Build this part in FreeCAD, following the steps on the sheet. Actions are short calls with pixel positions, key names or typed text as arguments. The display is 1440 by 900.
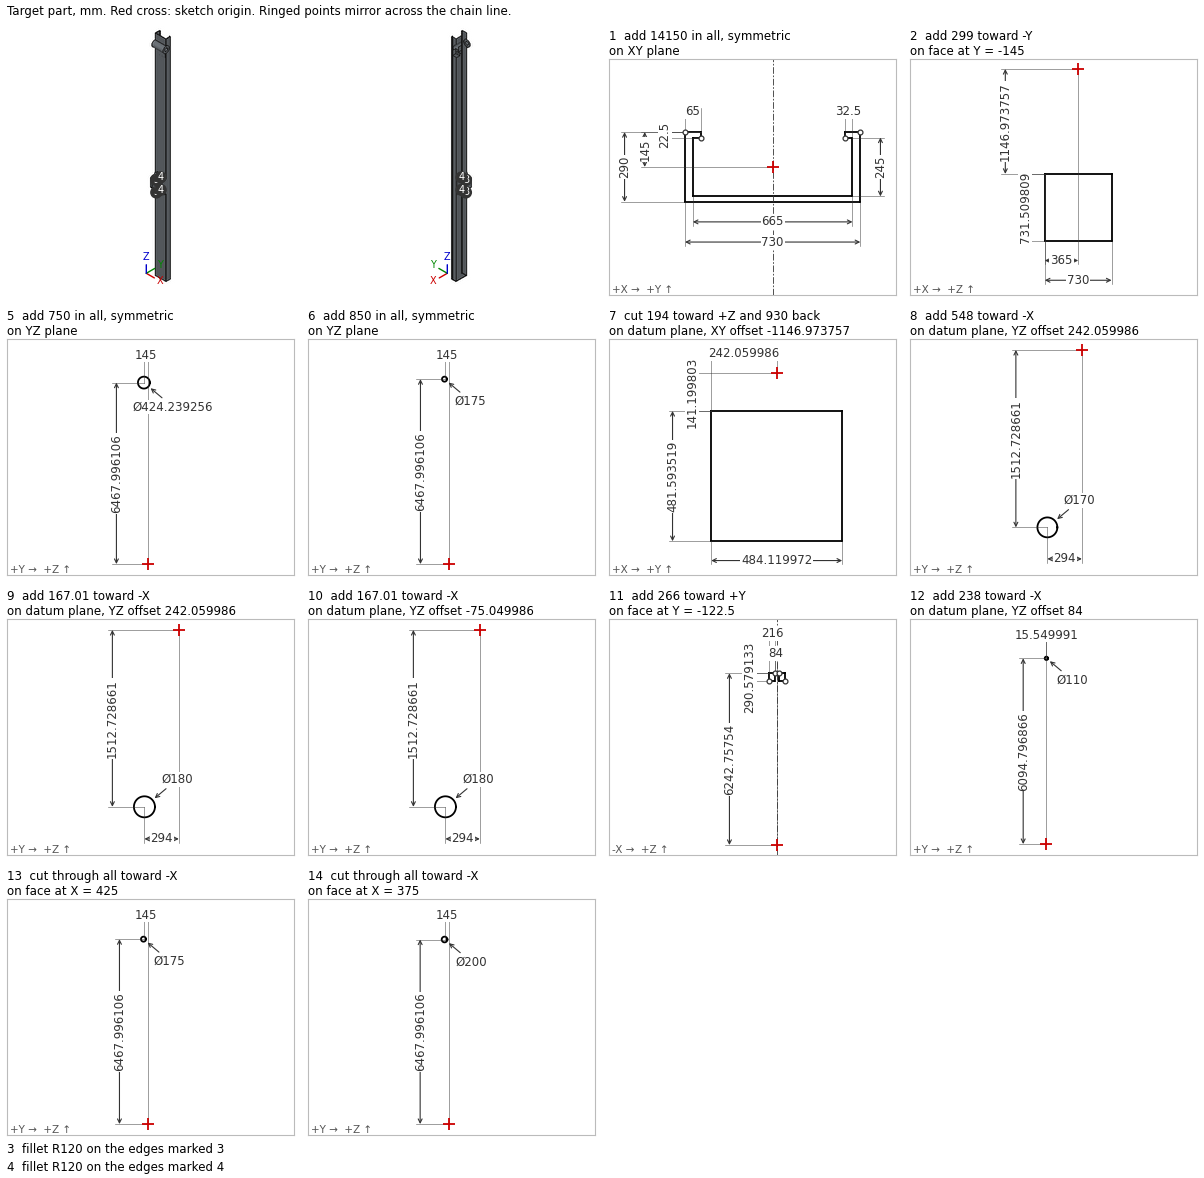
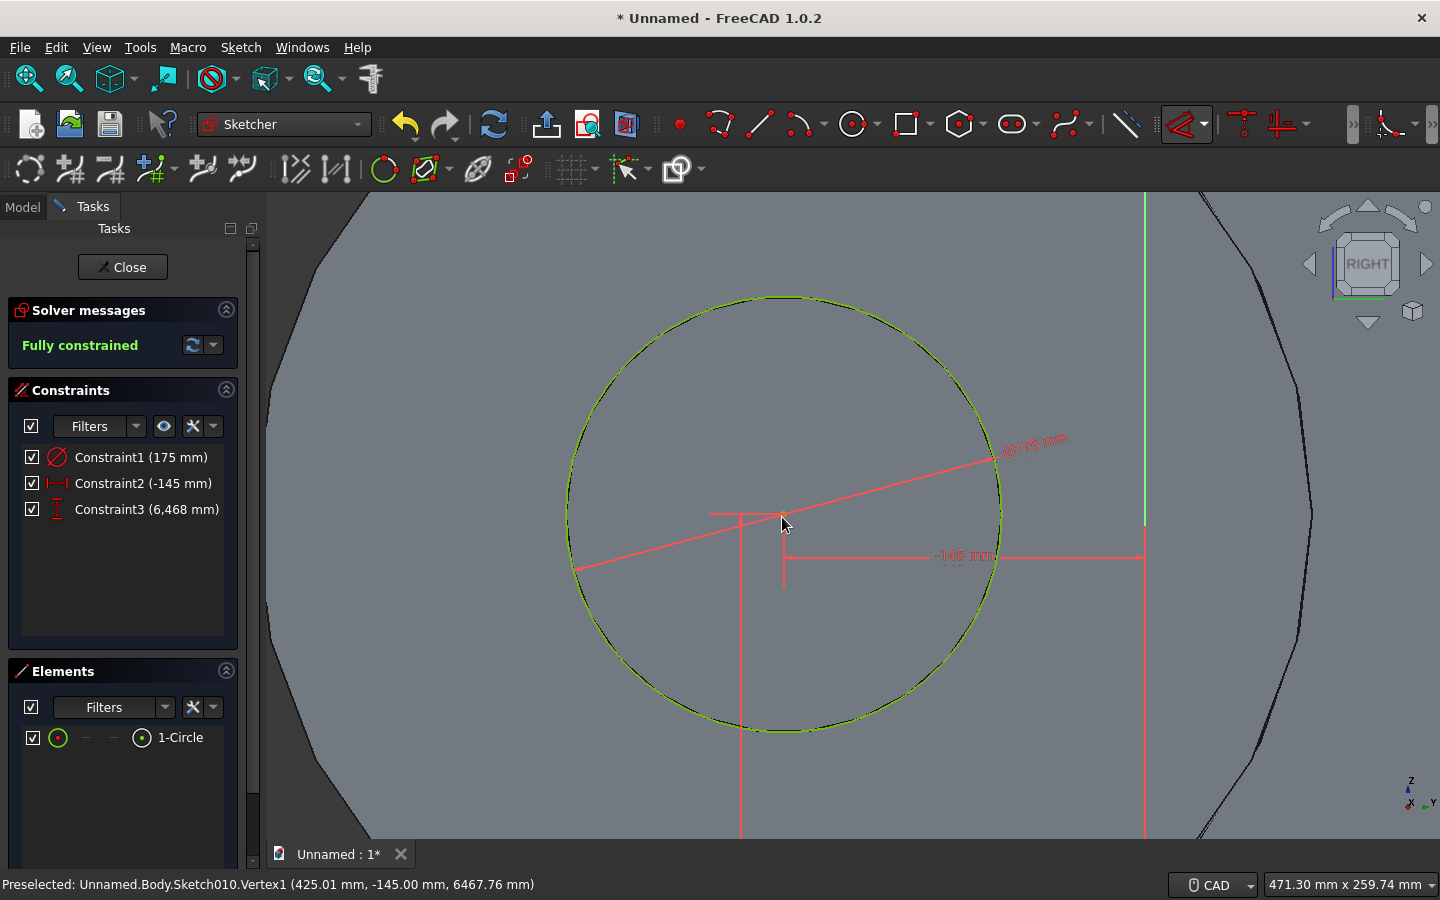
click(123, 267)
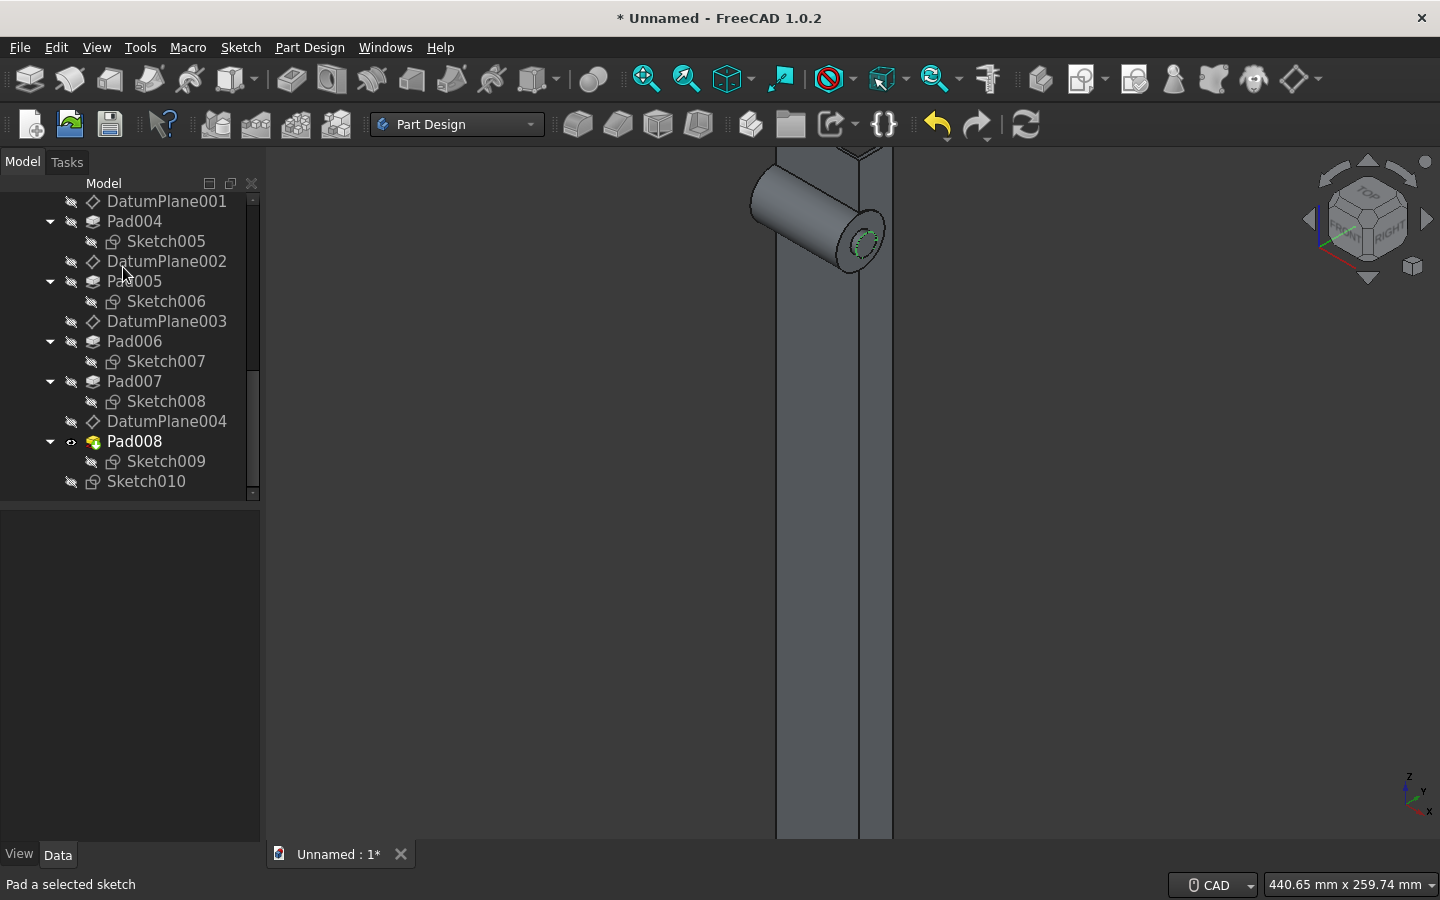
click(292, 80)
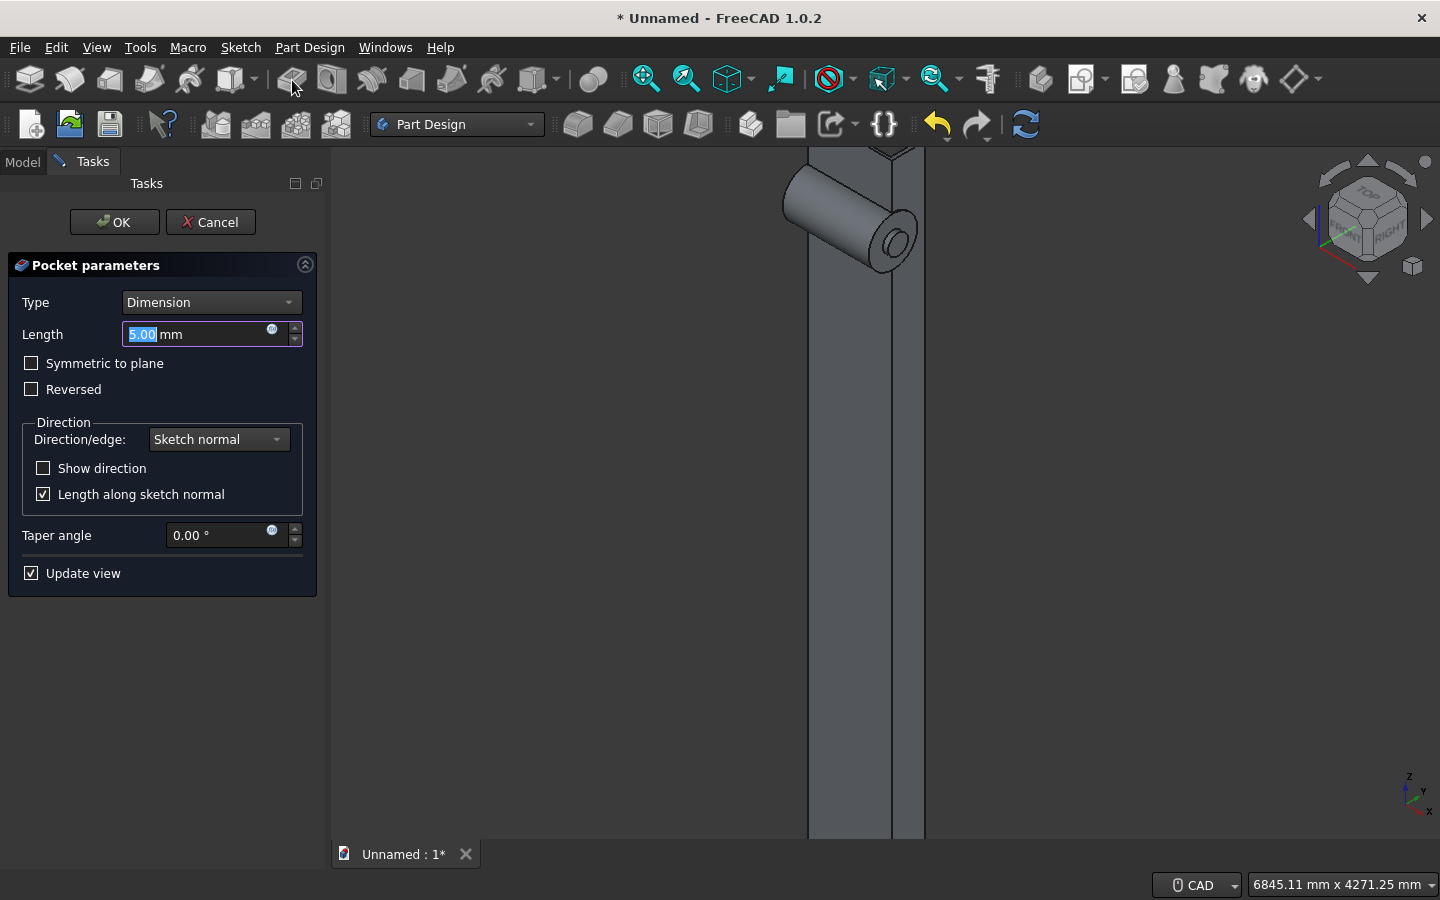
click(212, 302)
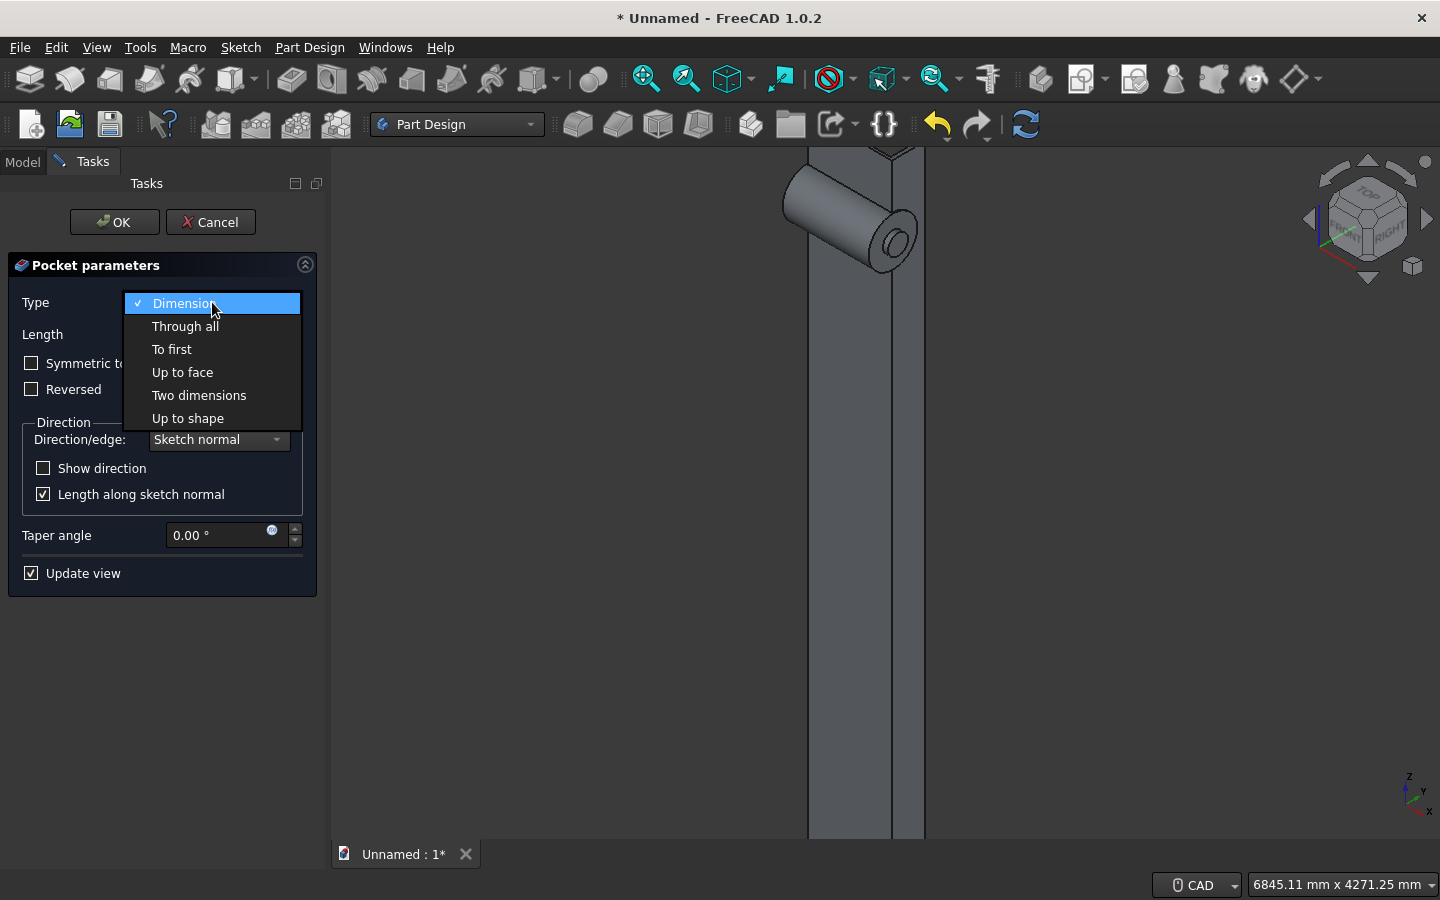
click(212, 326)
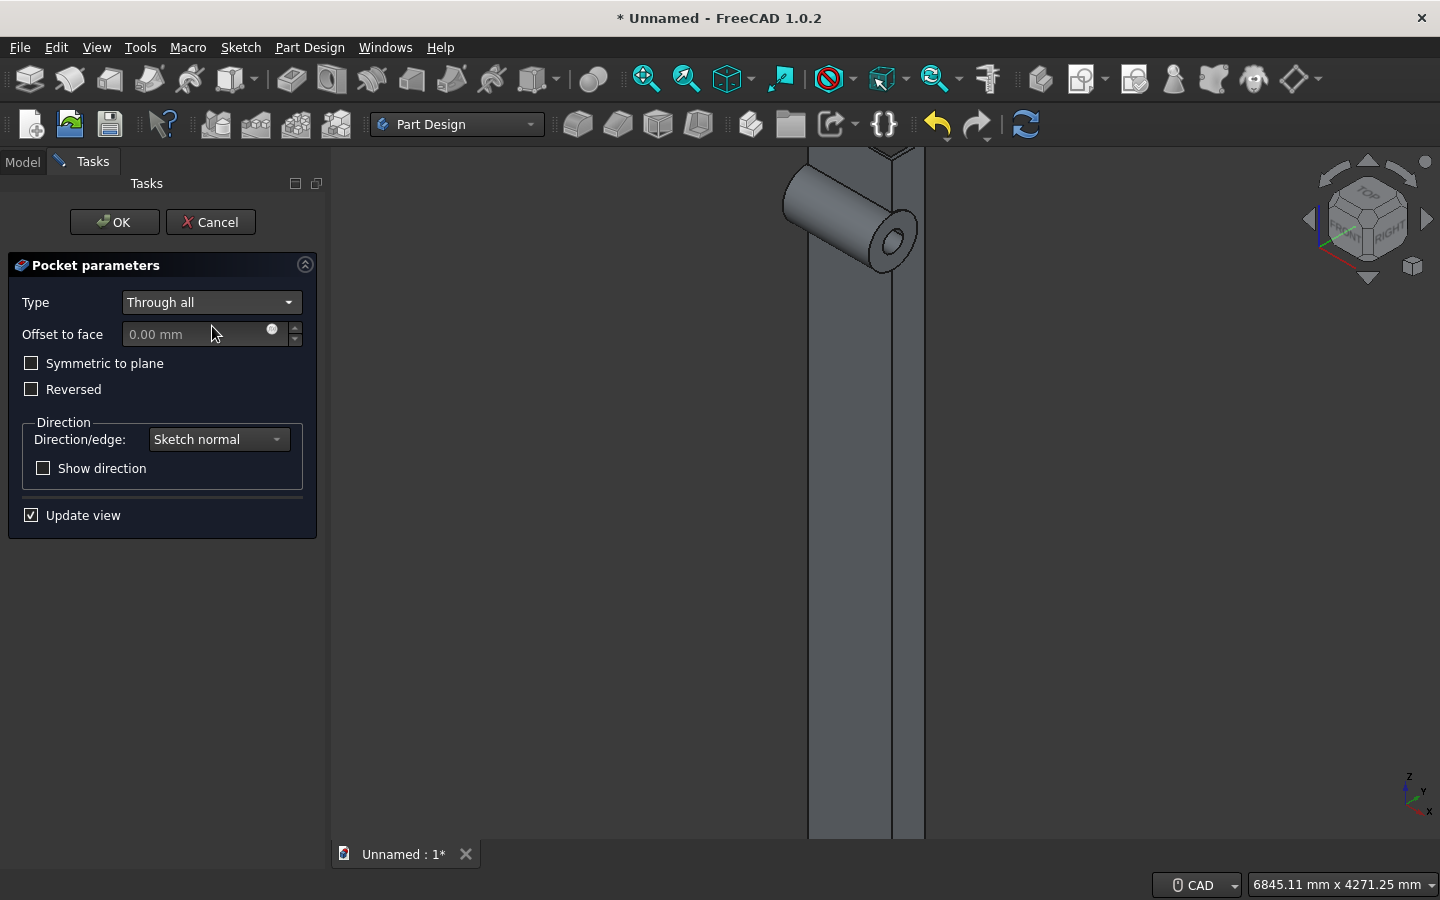
click(115, 222)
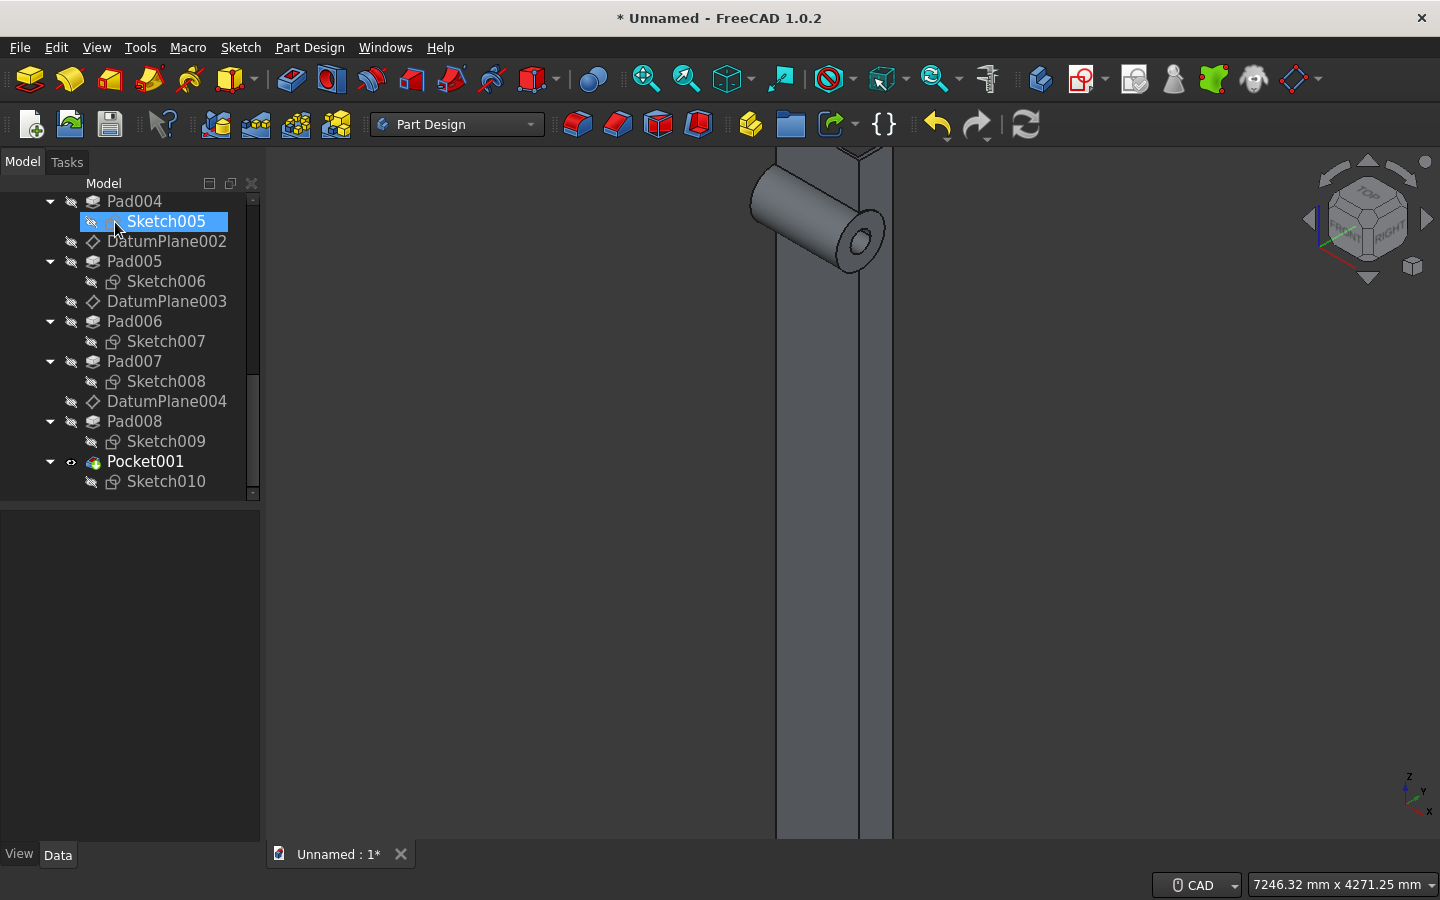
click(648, 80)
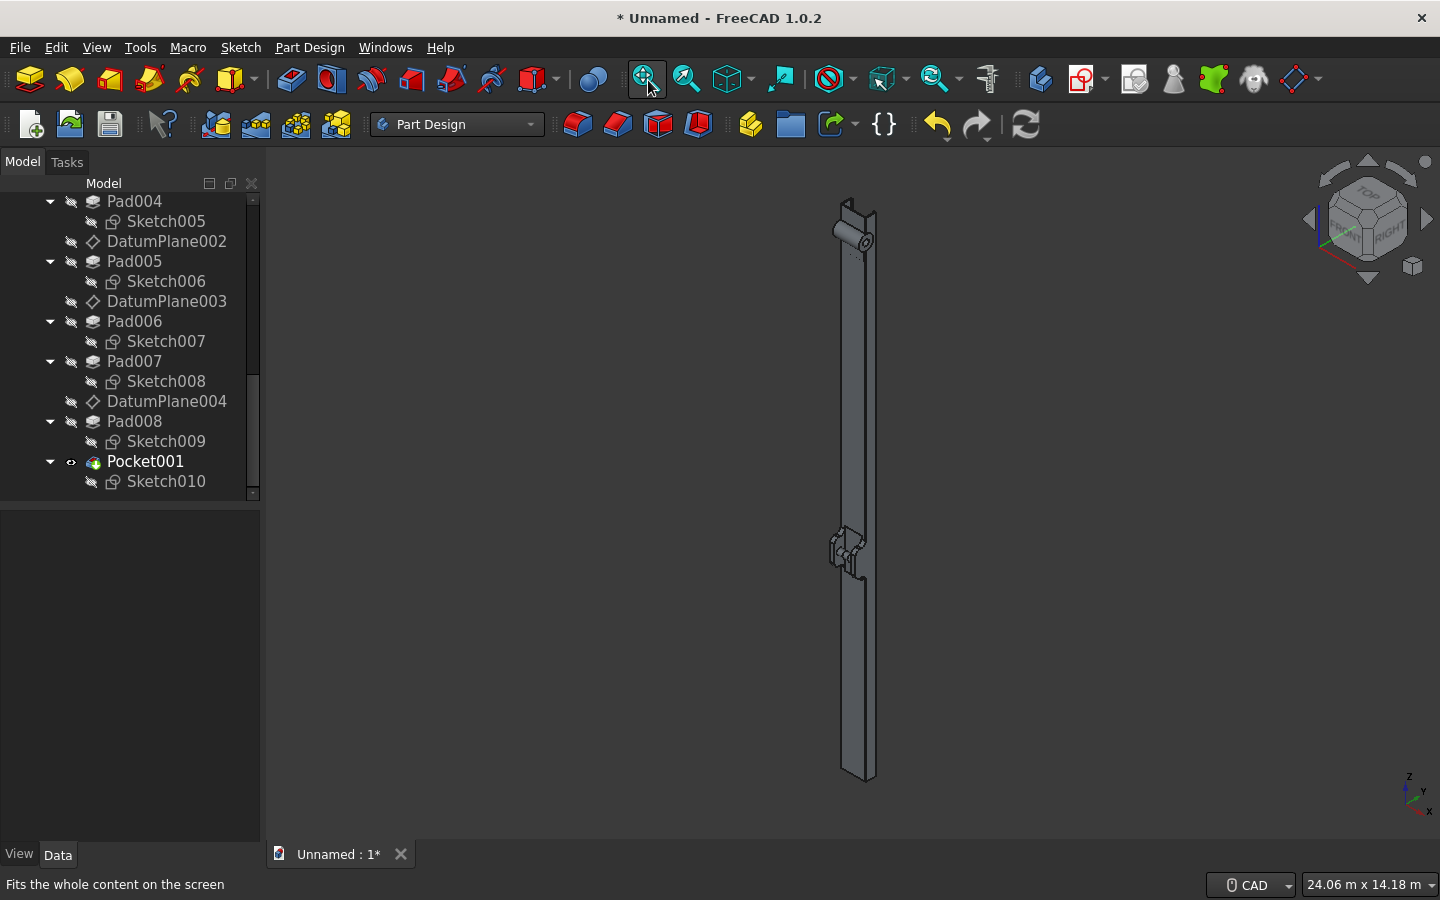
scroll(870, 237, up, 9)